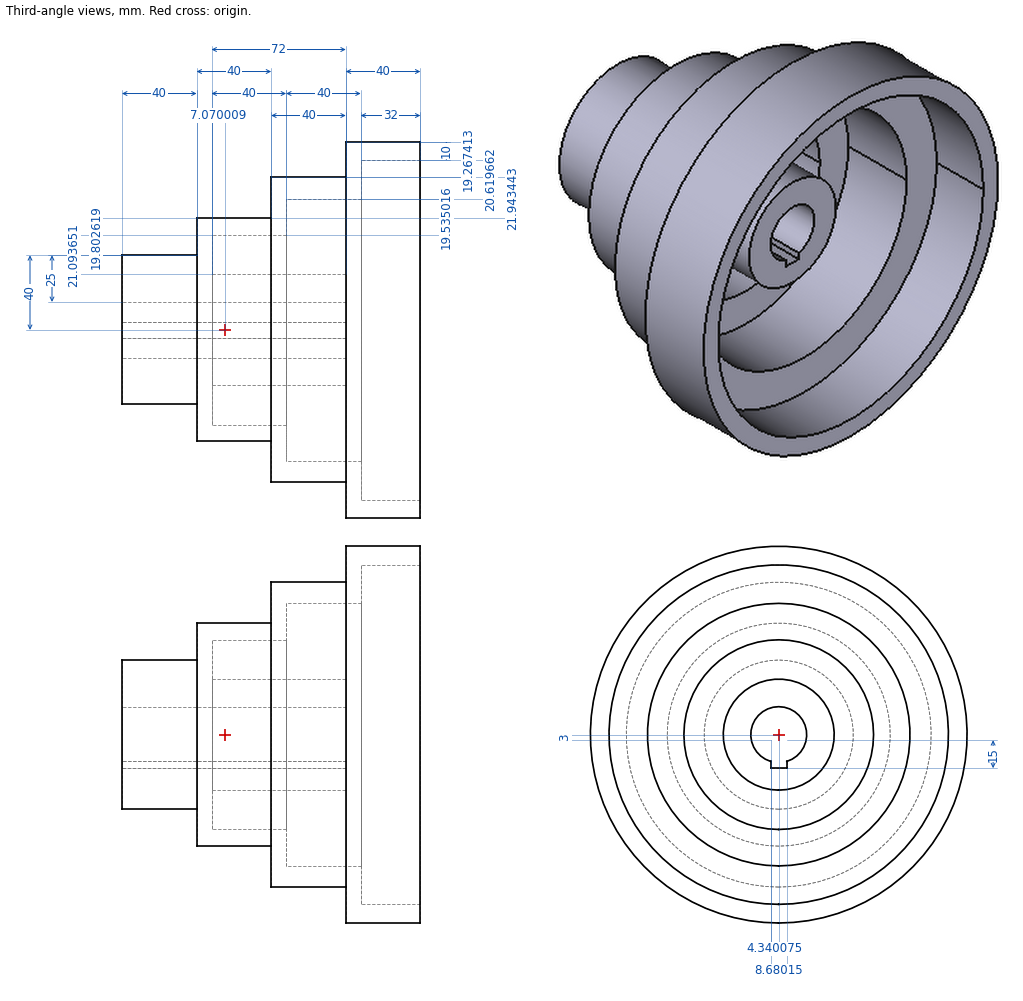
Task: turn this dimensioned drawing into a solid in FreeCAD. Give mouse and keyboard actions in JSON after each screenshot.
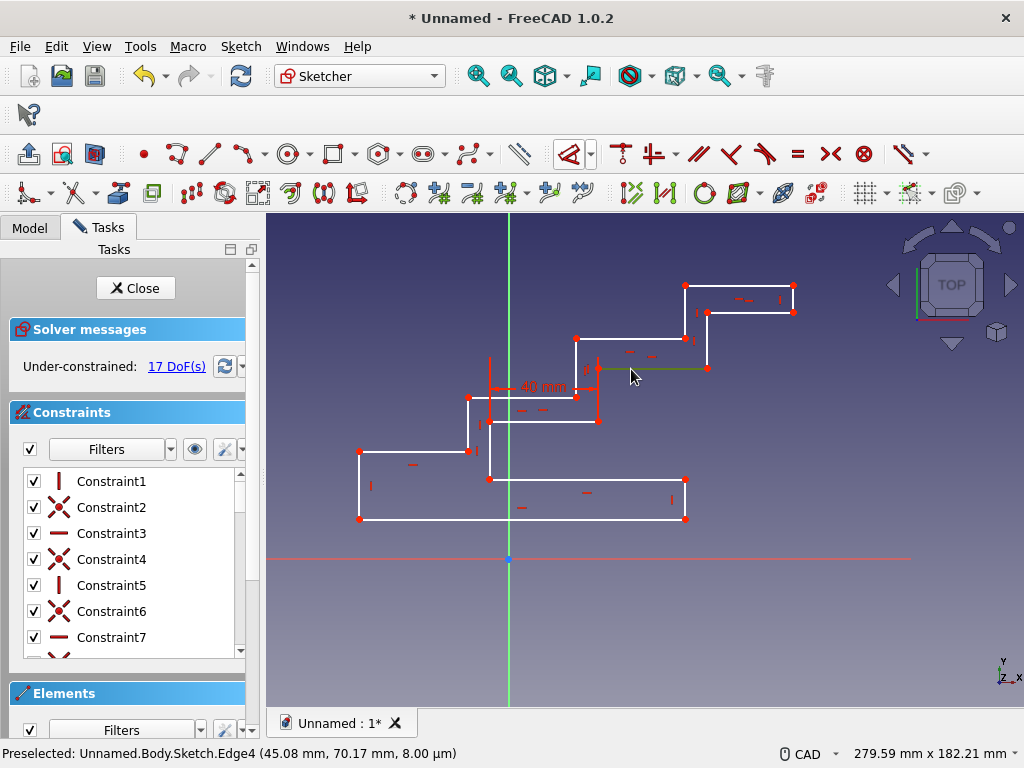
{"action": "left_click", "coordinate": [590, 154]}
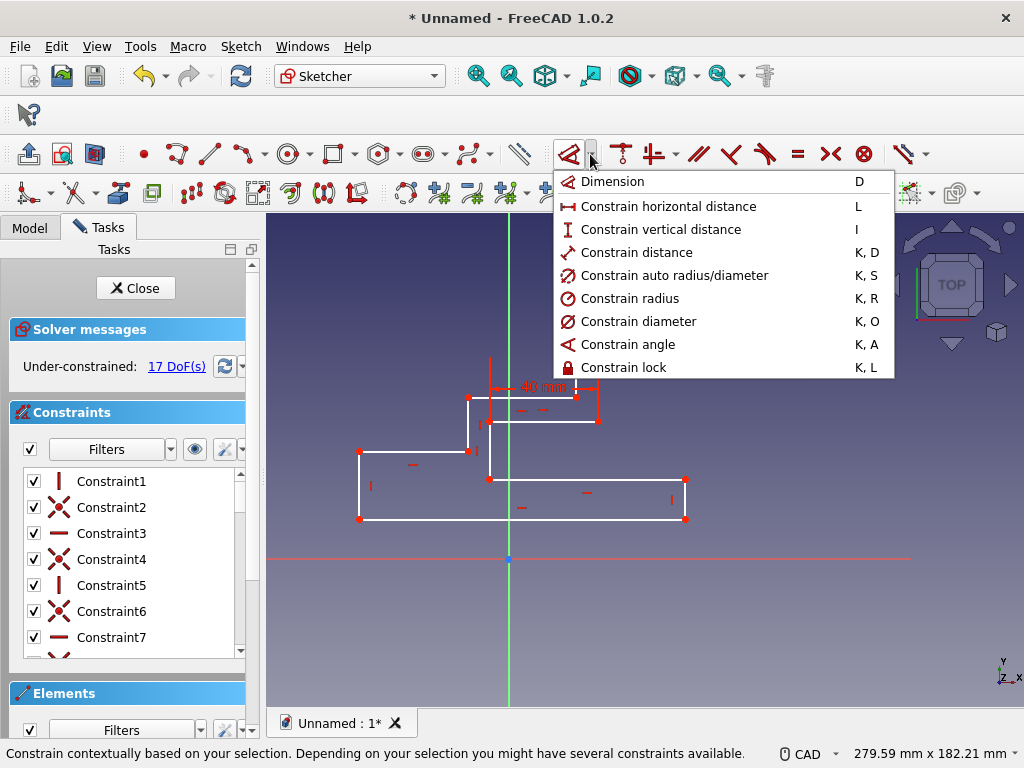
{"action": "left_click", "coordinate": [724, 206]}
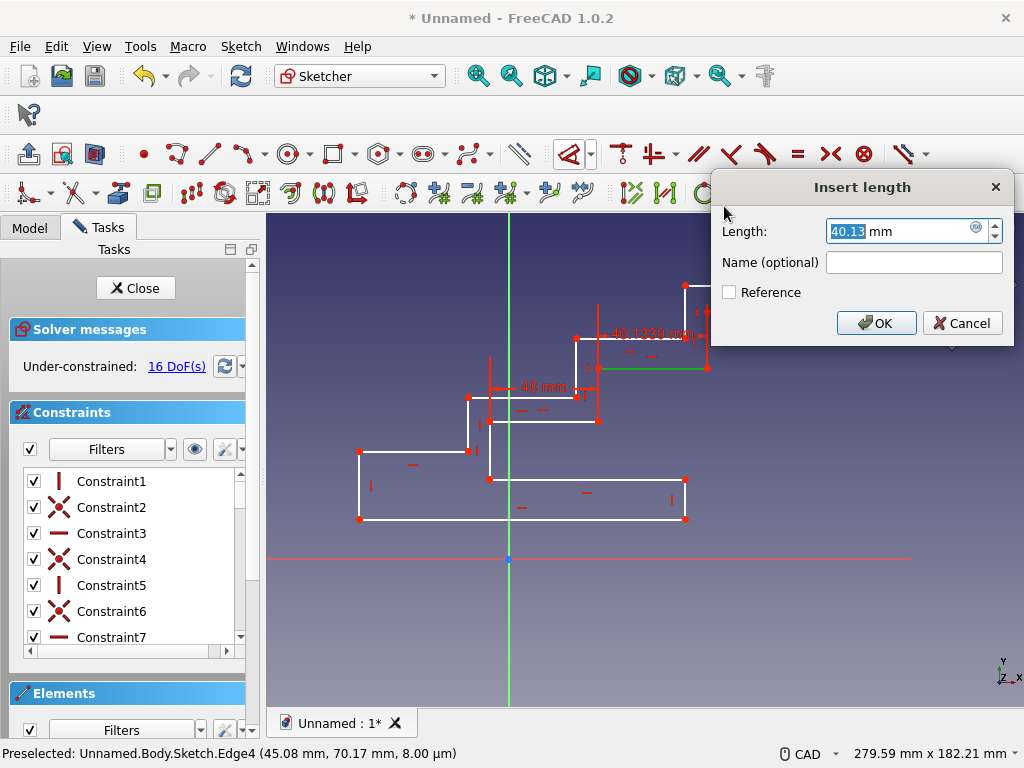
{"action": "type", "text": "40"}
{"action": "key", "text": "Return"}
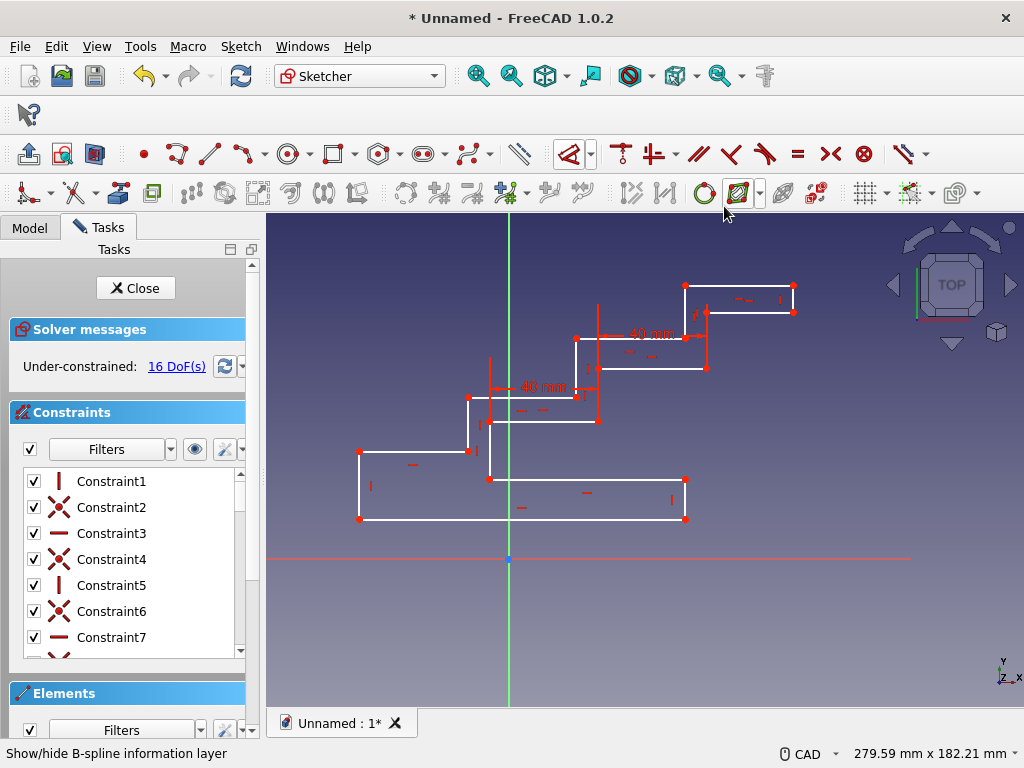
{"action": "left_click", "coordinate": [733, 313]}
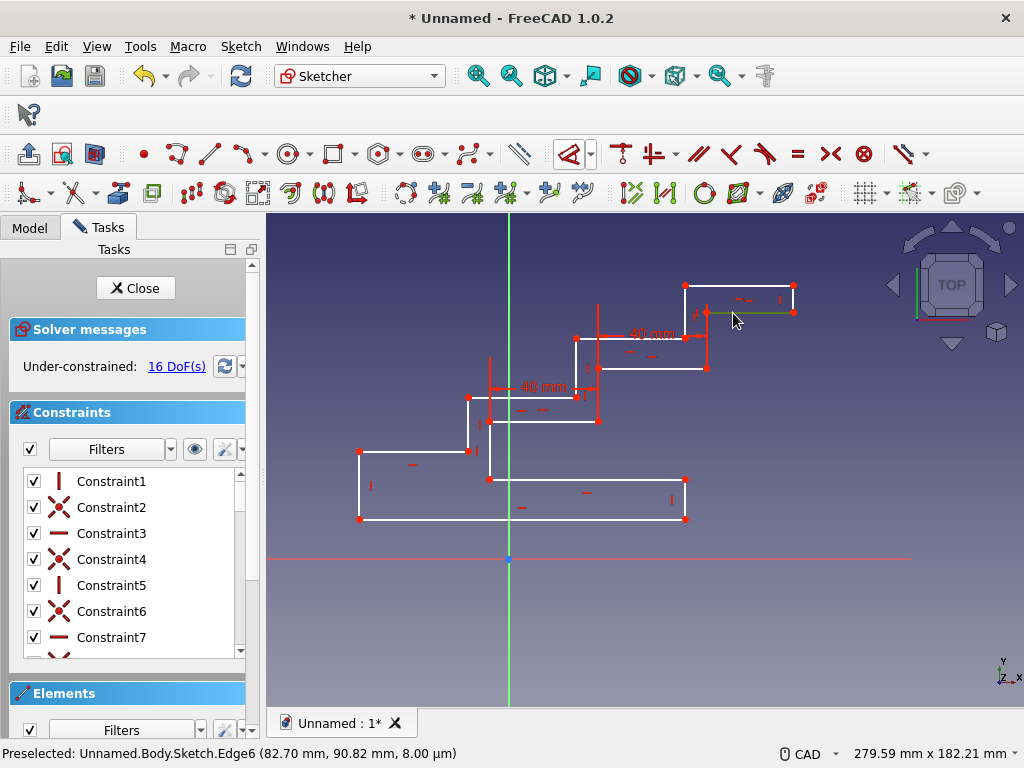
{"action": "left_click", "coordinate": [590, 154]}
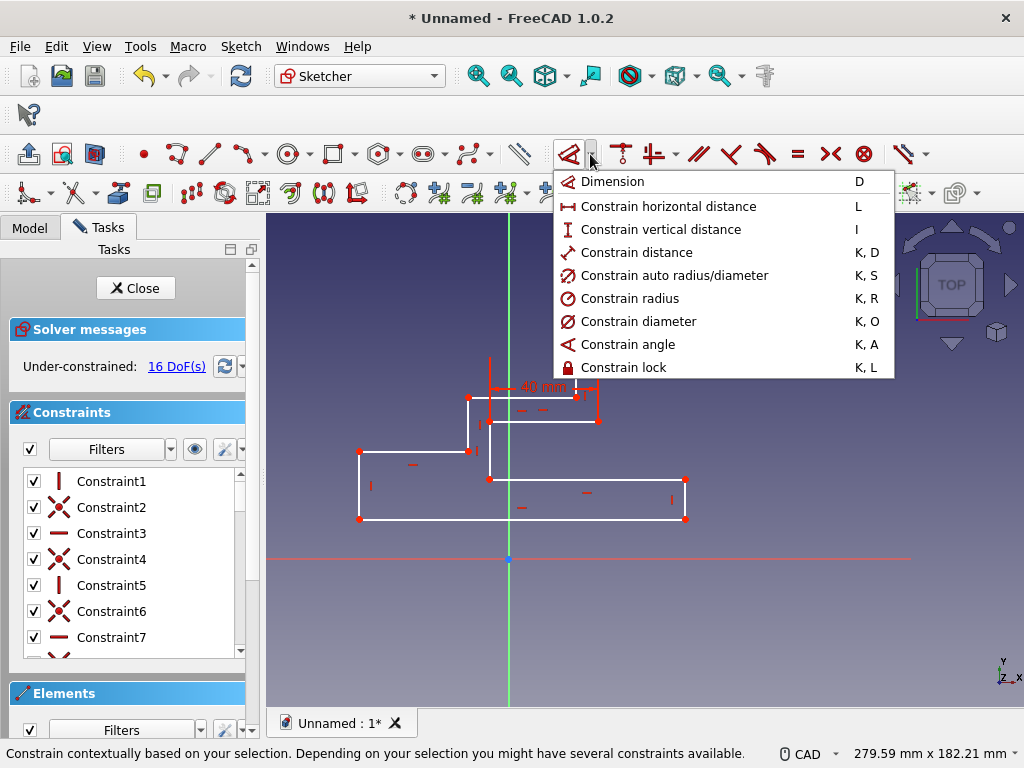
{"action": "left_click", "coordinate": [724, 206]}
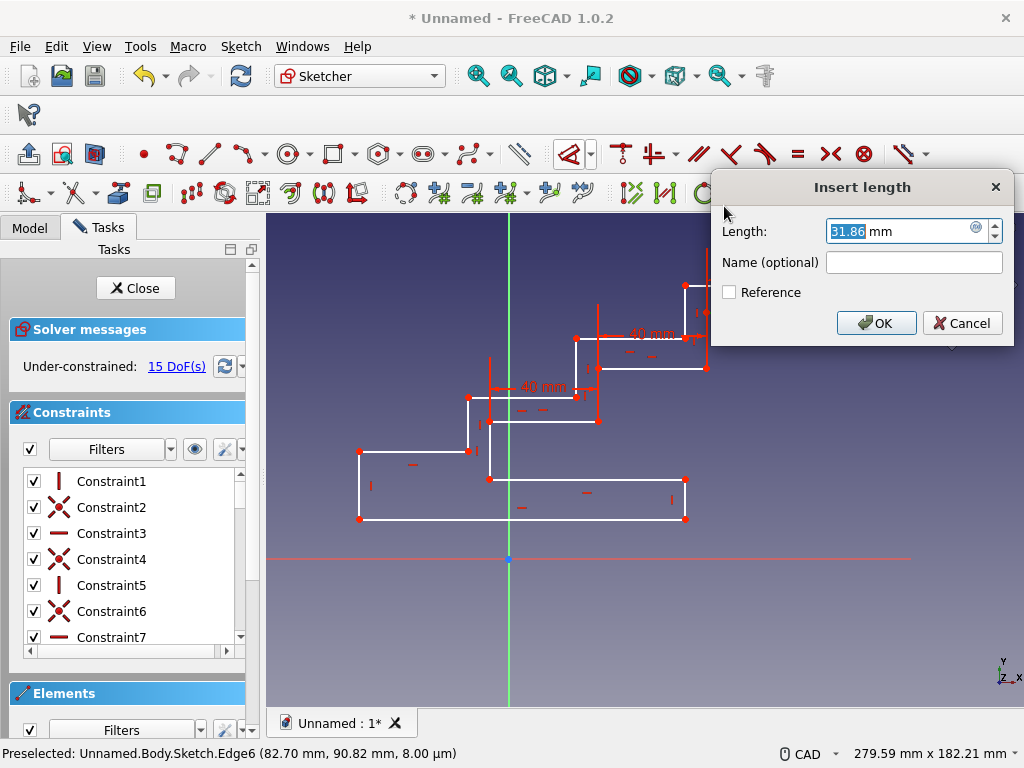
{"action": "type", "text": "32"}
{"action": "key", "text": "Return"}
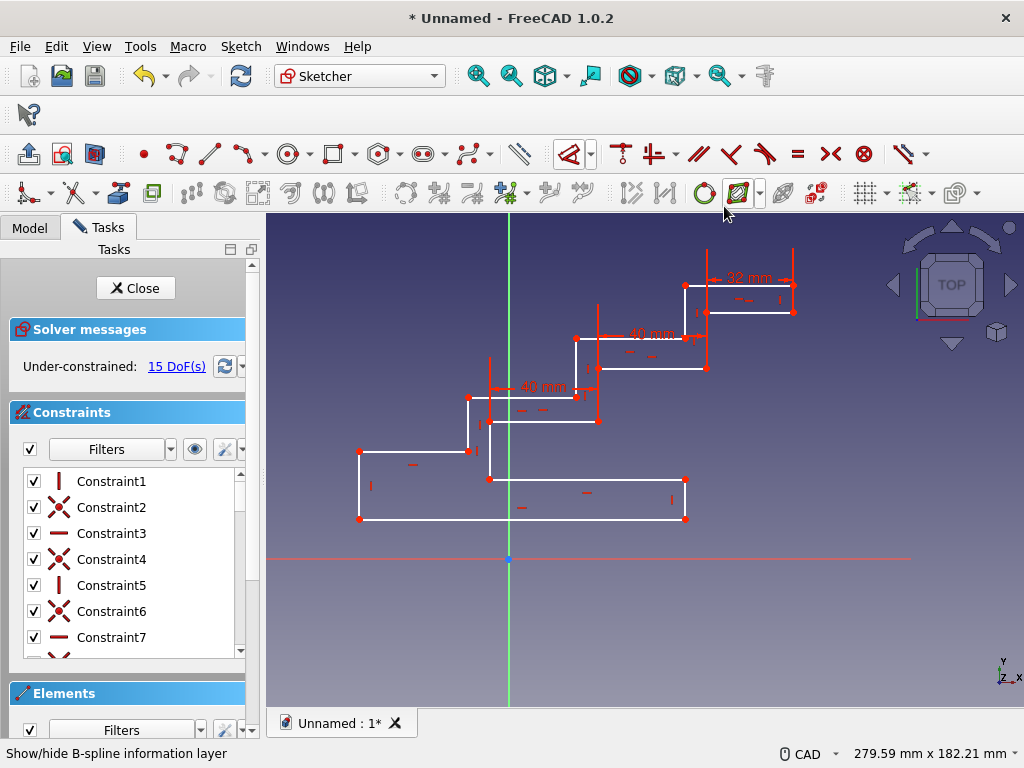
{"action": "scroll", "coordinate": [793, 302], "scroll_direction": "up", "scroll_amount": 2}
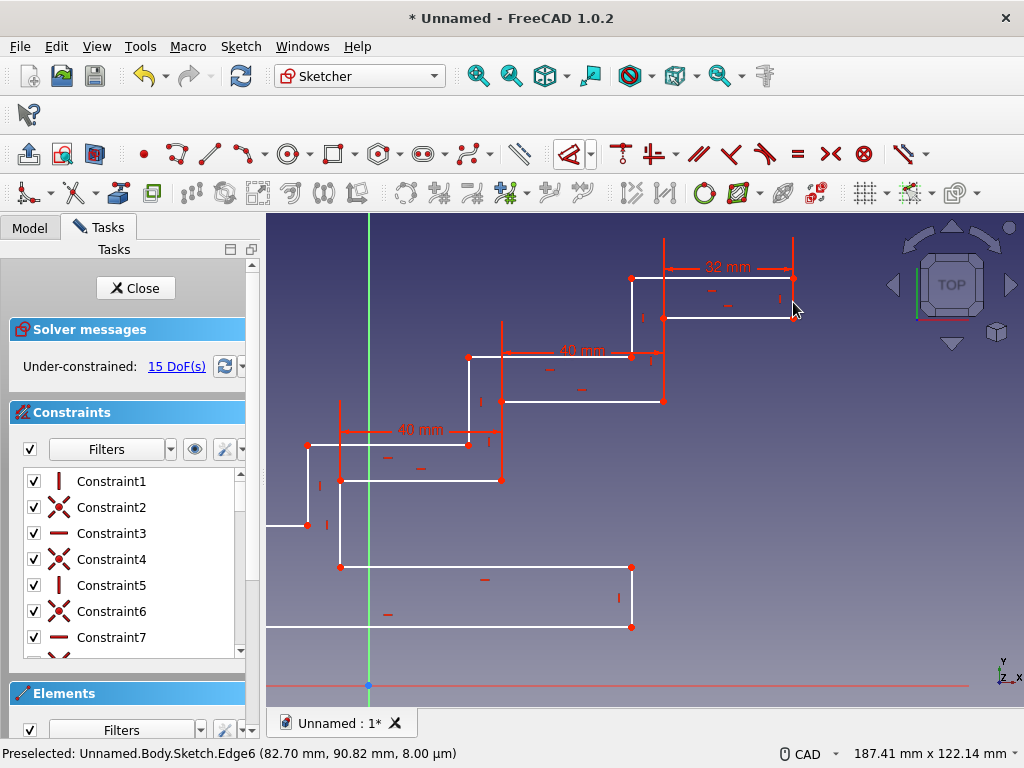
{"action": "left_click", "coordinate": [793, 302]}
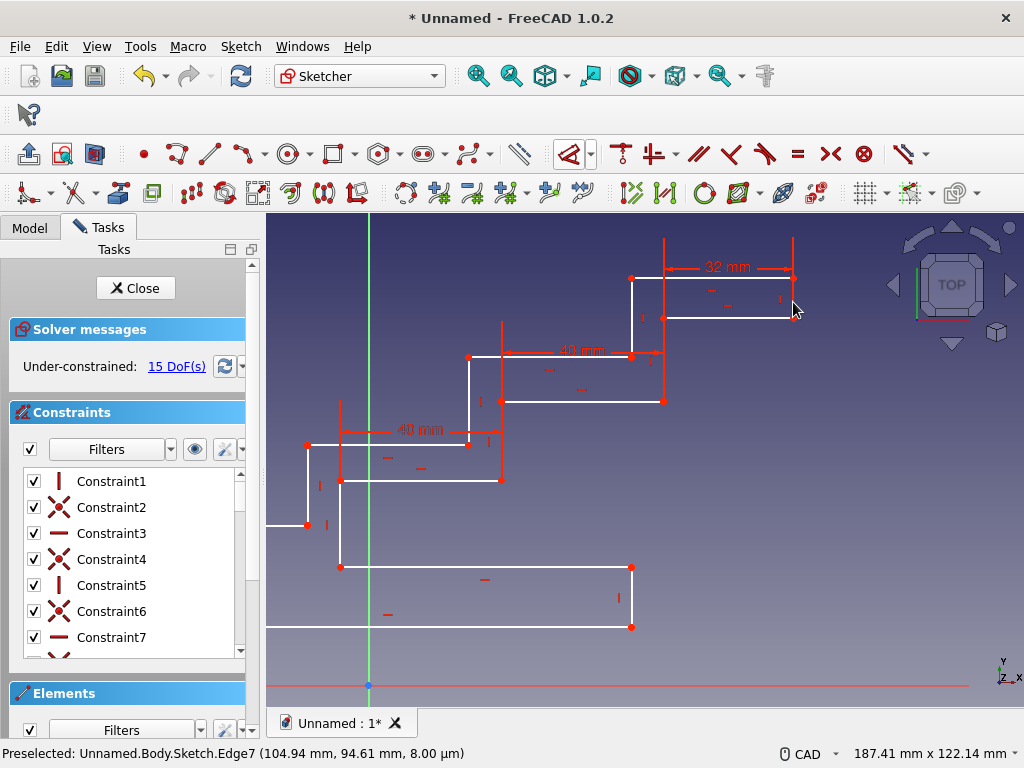
{"action": "key", "text": "i"}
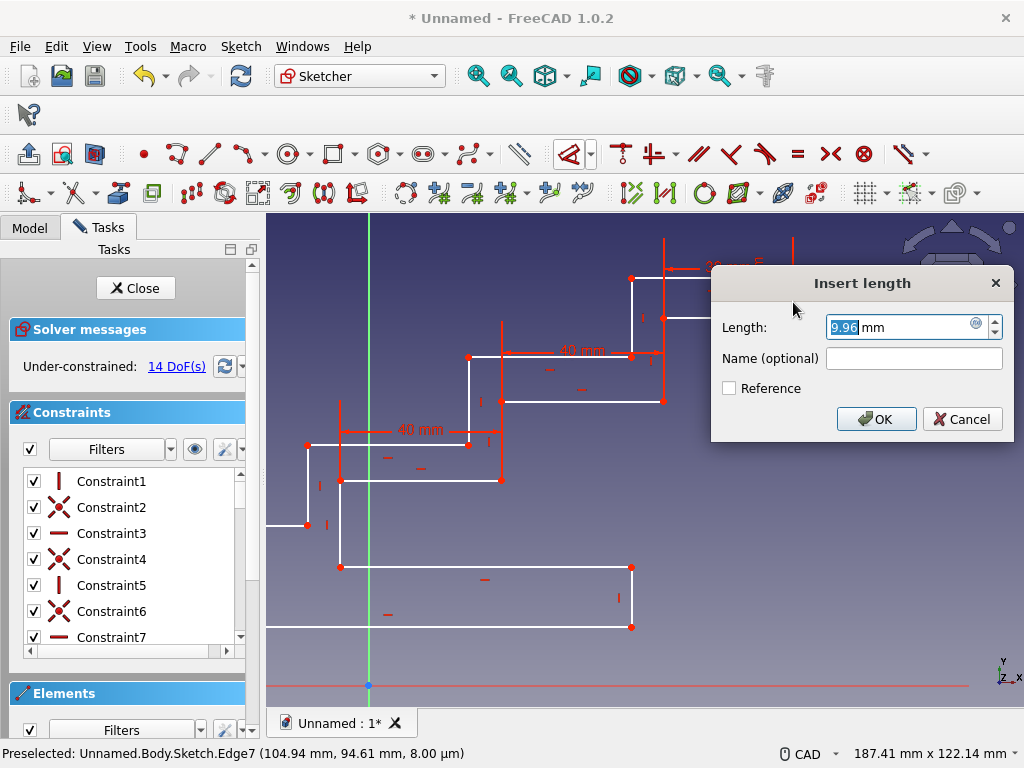
{"action": "type", "text": "10"}
{"action": "key", "text": "Return"}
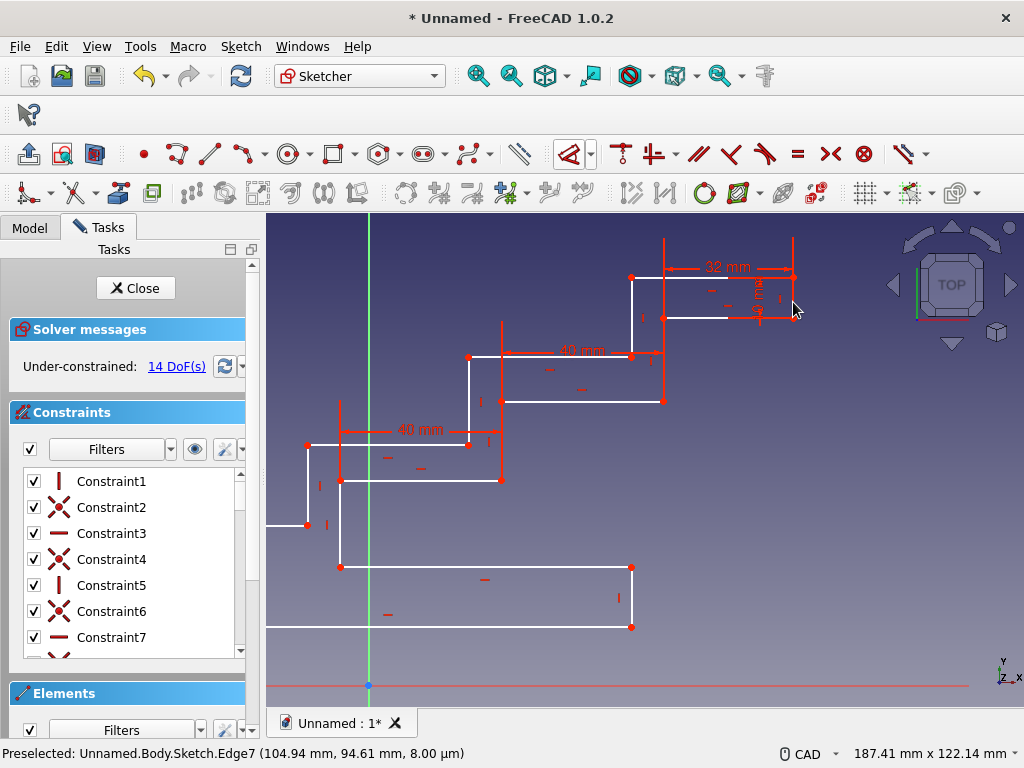
{"action": "left_click", "coordinate": [745, 278]}